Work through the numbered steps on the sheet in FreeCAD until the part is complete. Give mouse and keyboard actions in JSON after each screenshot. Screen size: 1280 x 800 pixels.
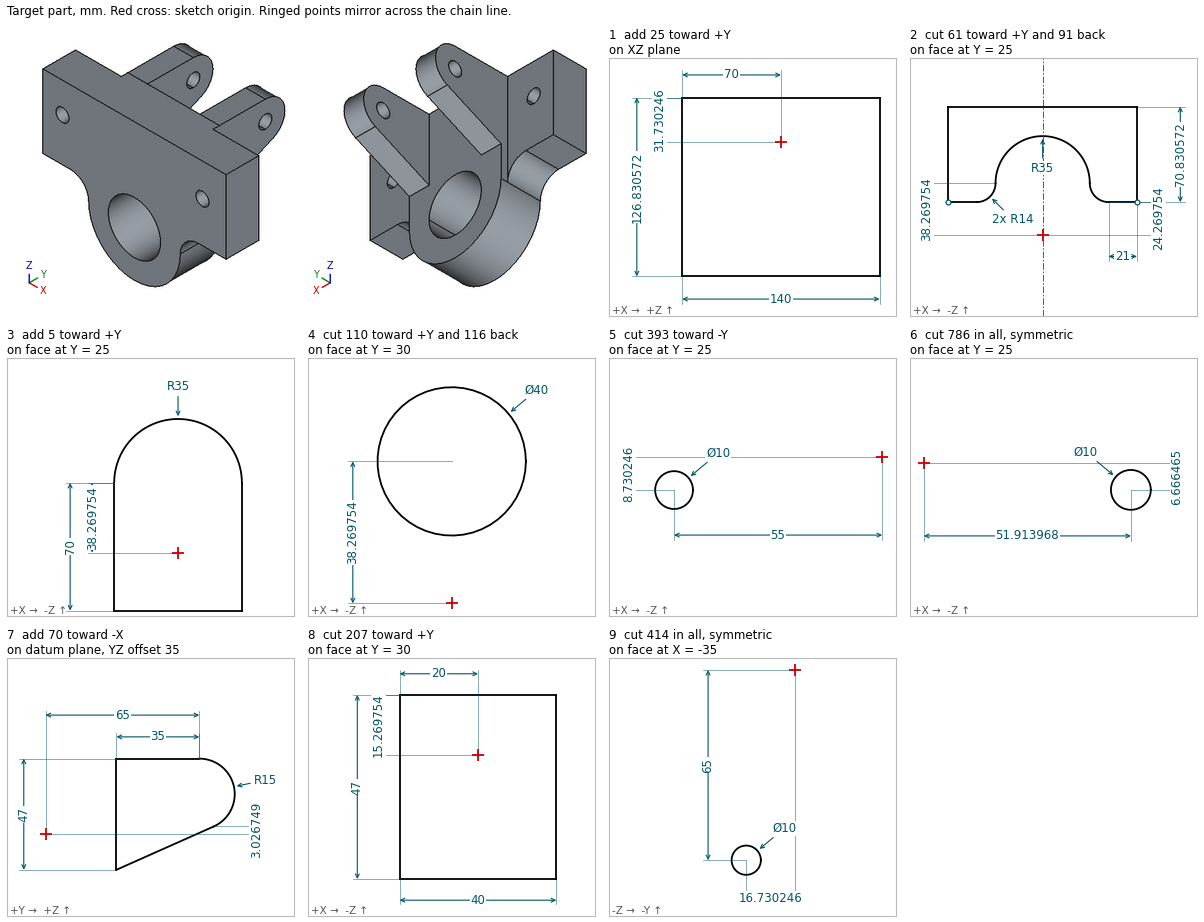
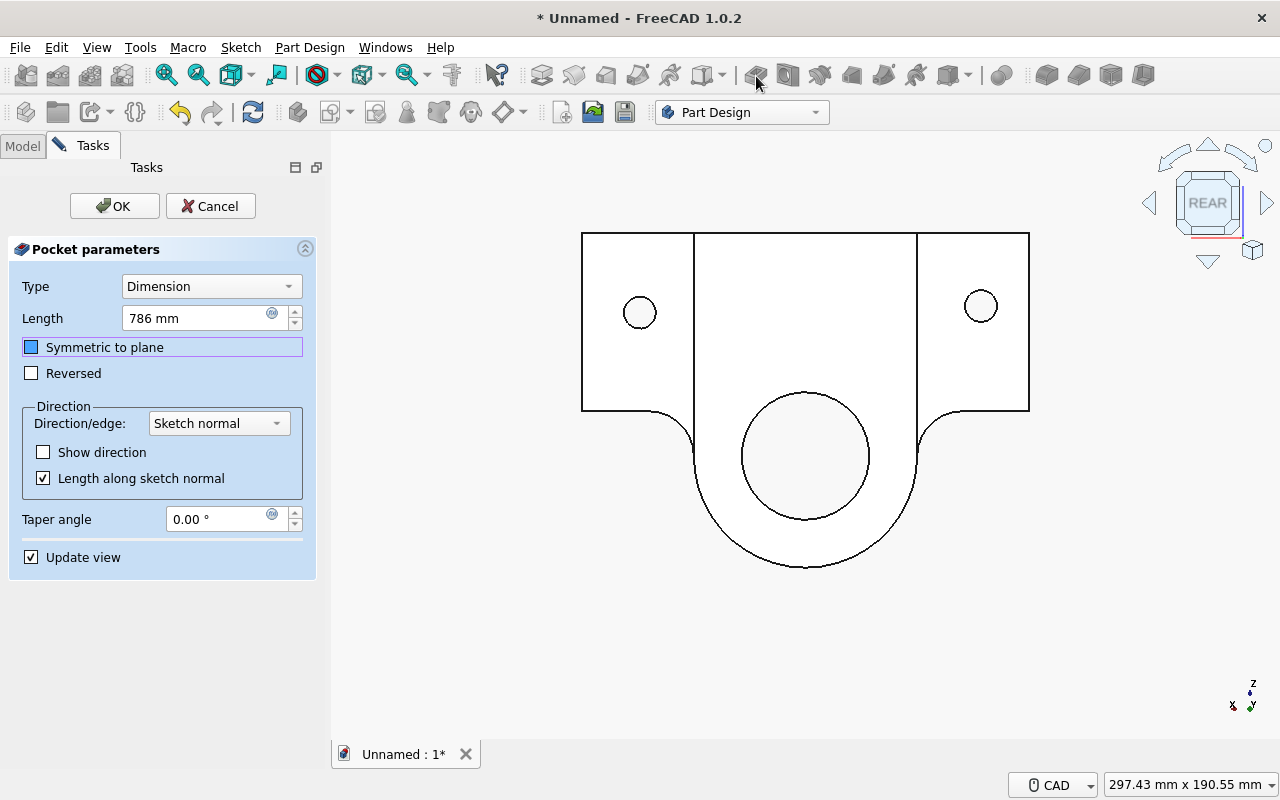
{"action": "left_click", "coordinate": [30, 347]}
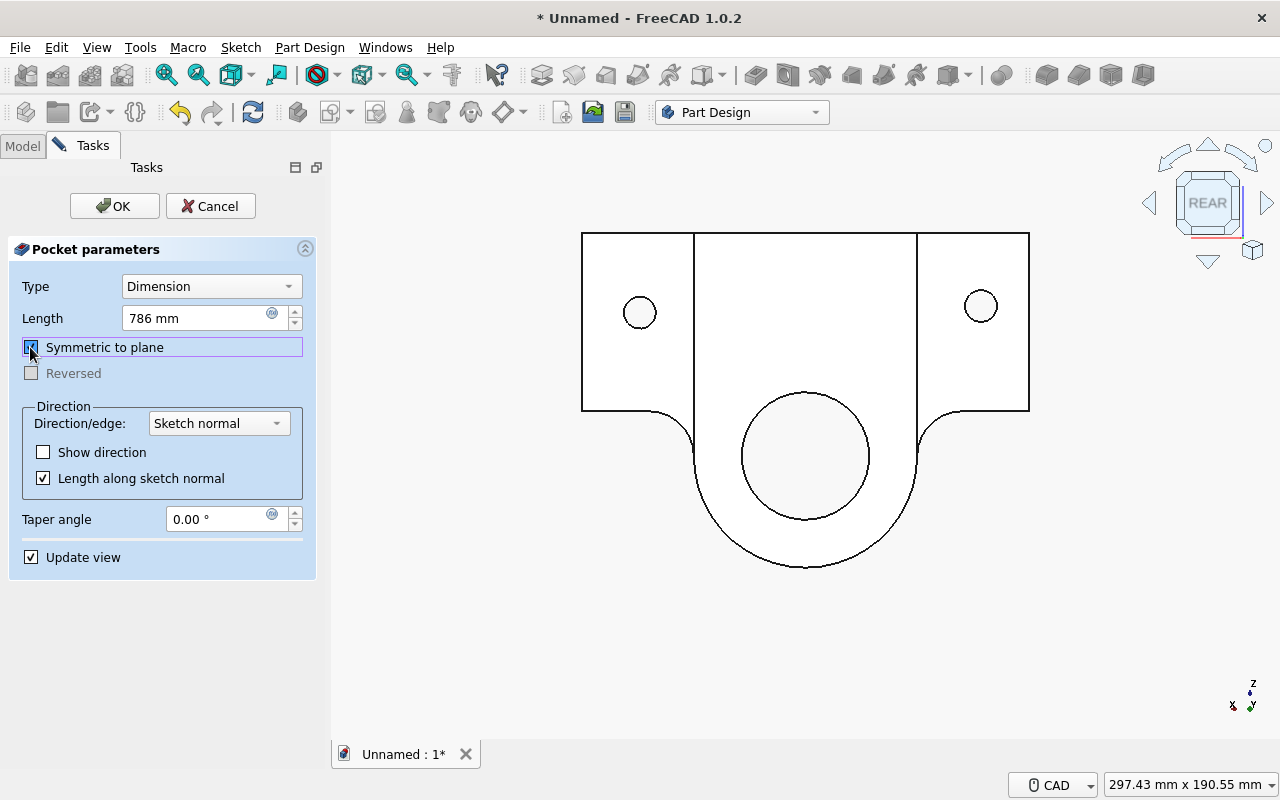
{"action": "left_click", "coordinate": [115, 206]}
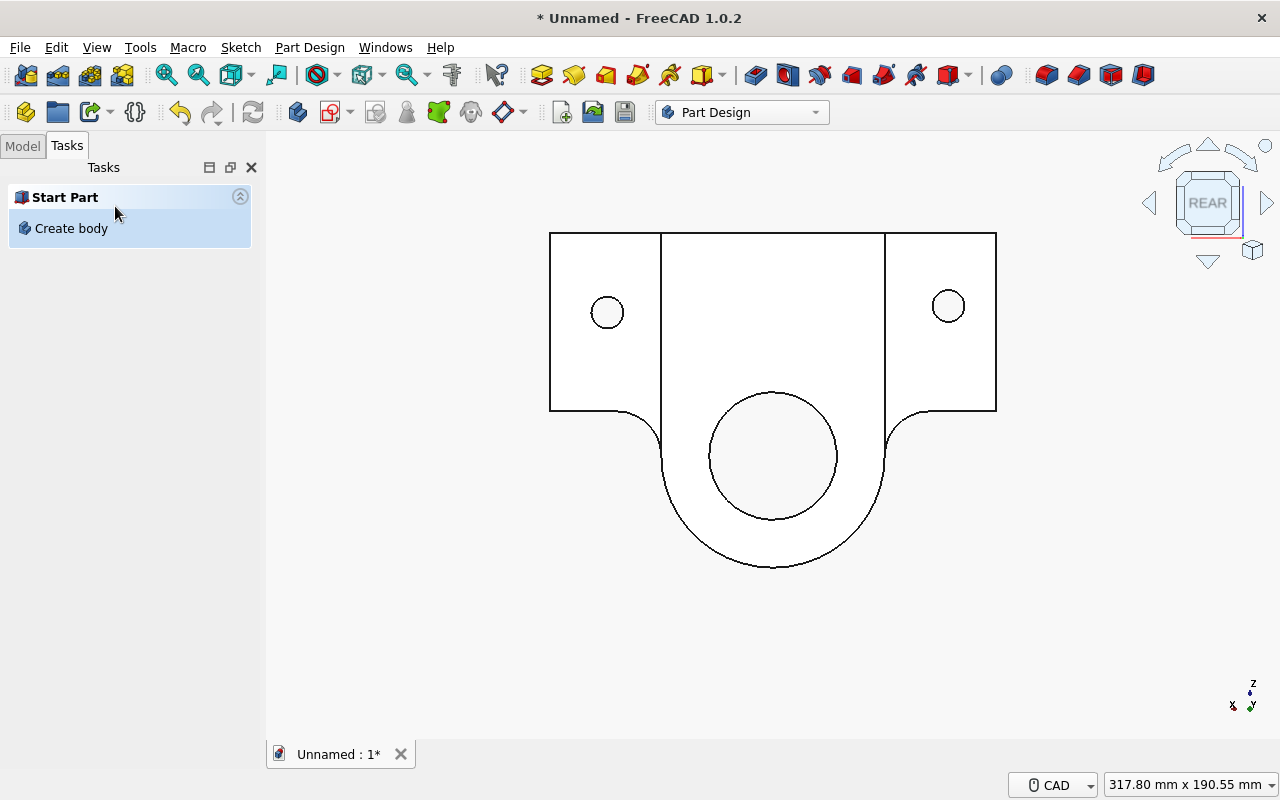
{"action": "key", "text": "0"}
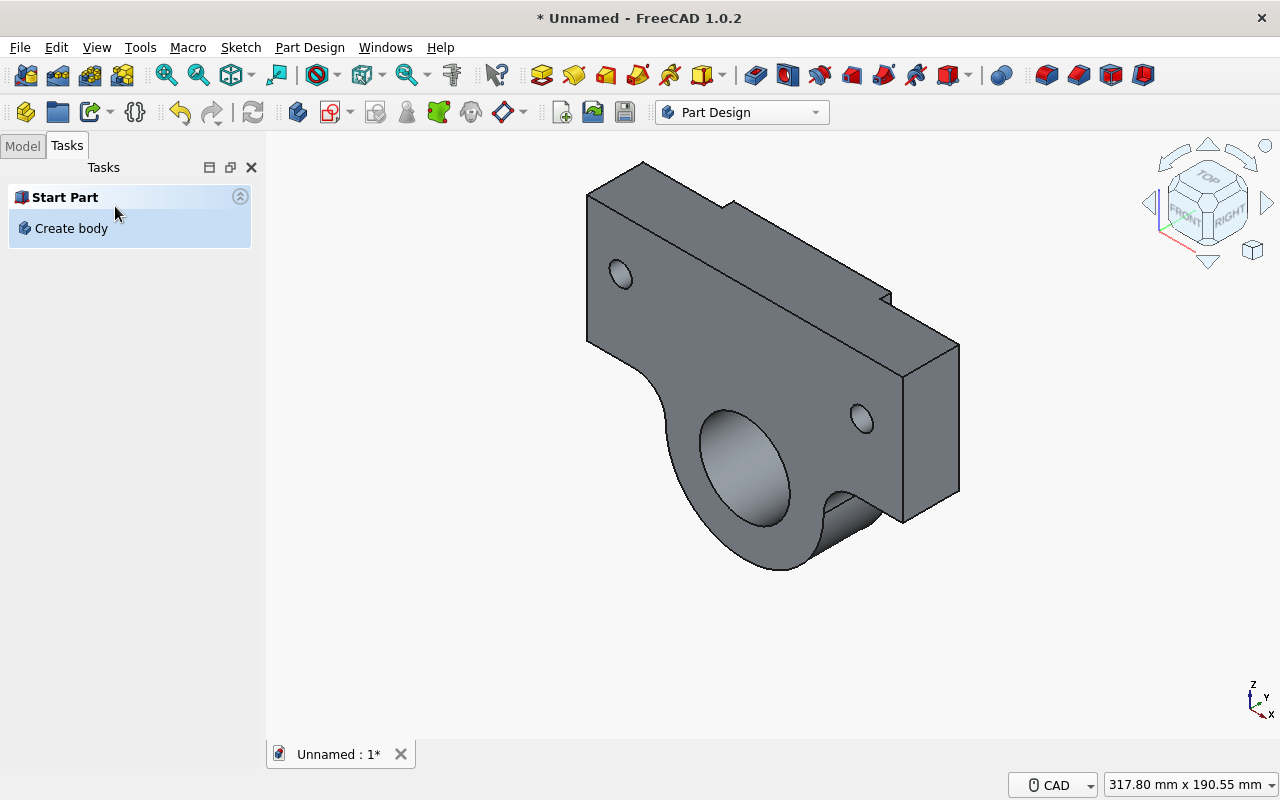
{"action": "key", "text": "3"}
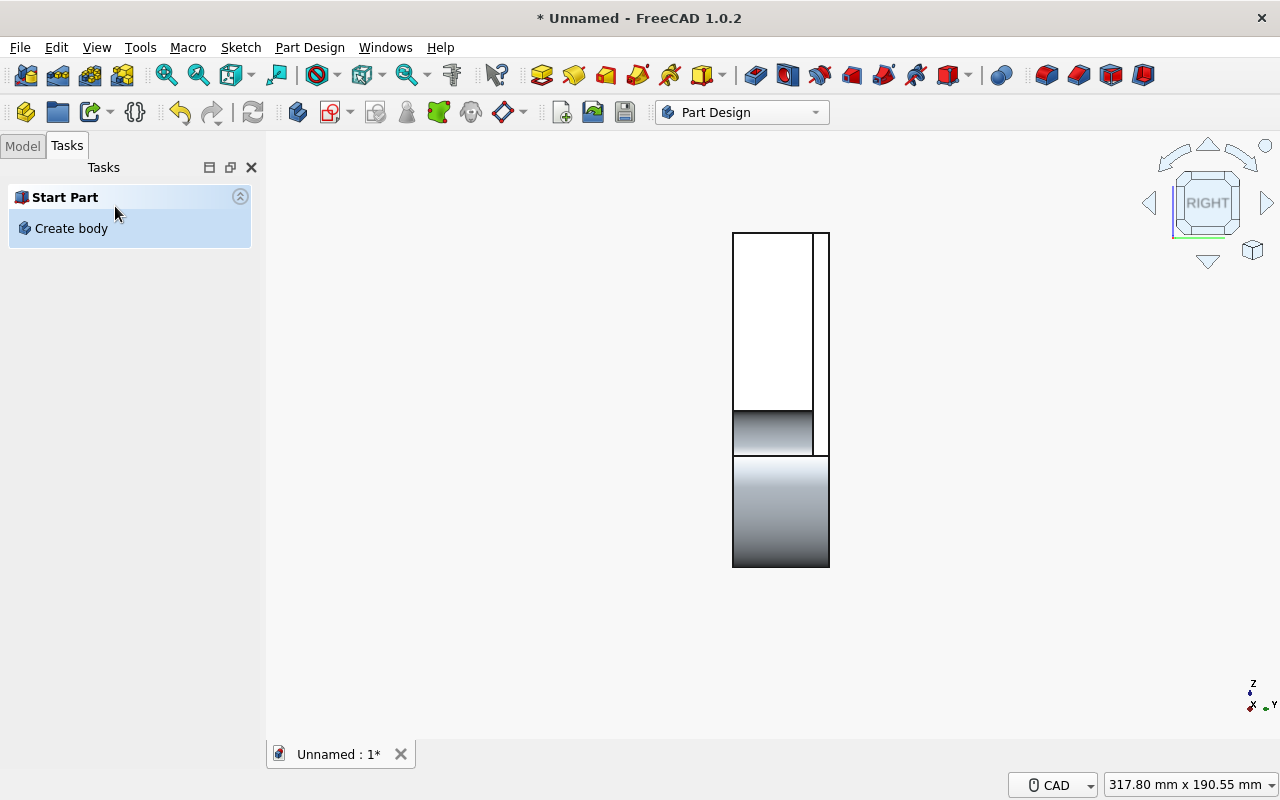
{"action": "key", "text": "2"}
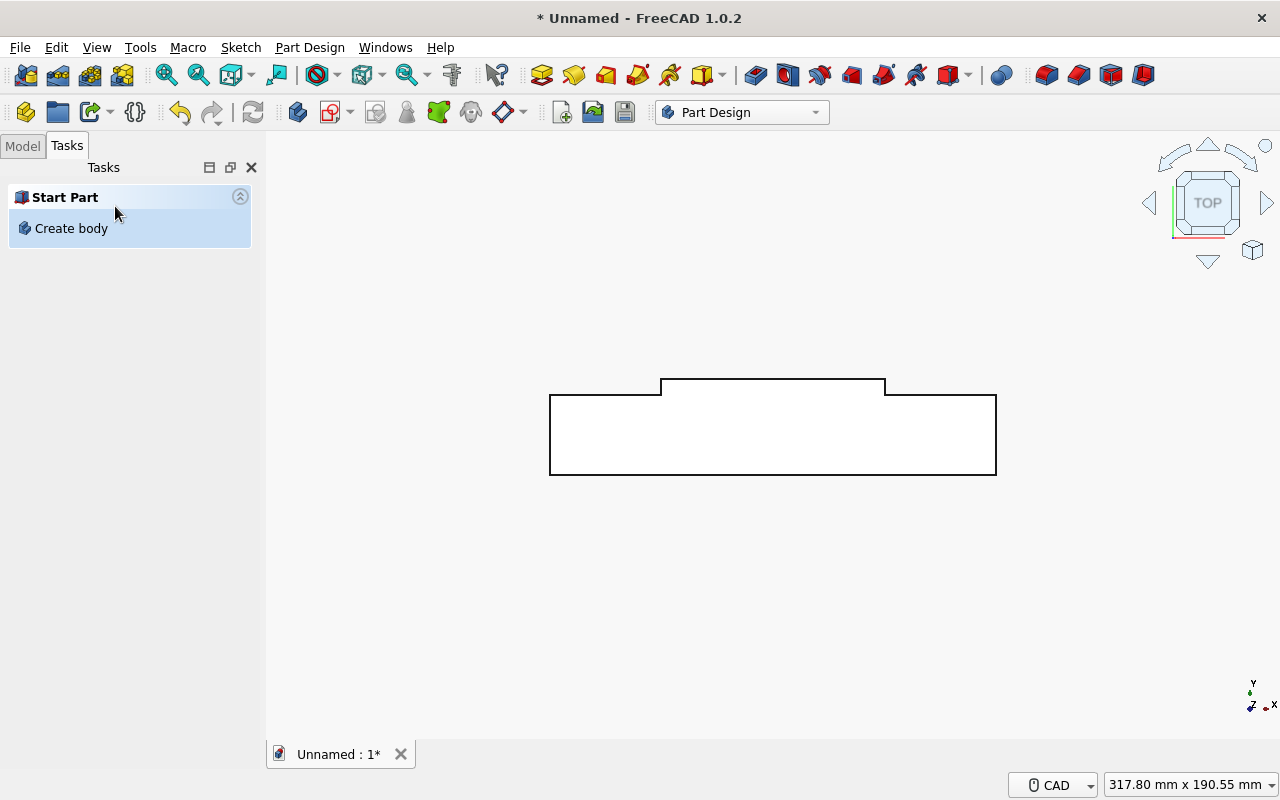
{"action": "left_click", "coordinate": [168, 76]}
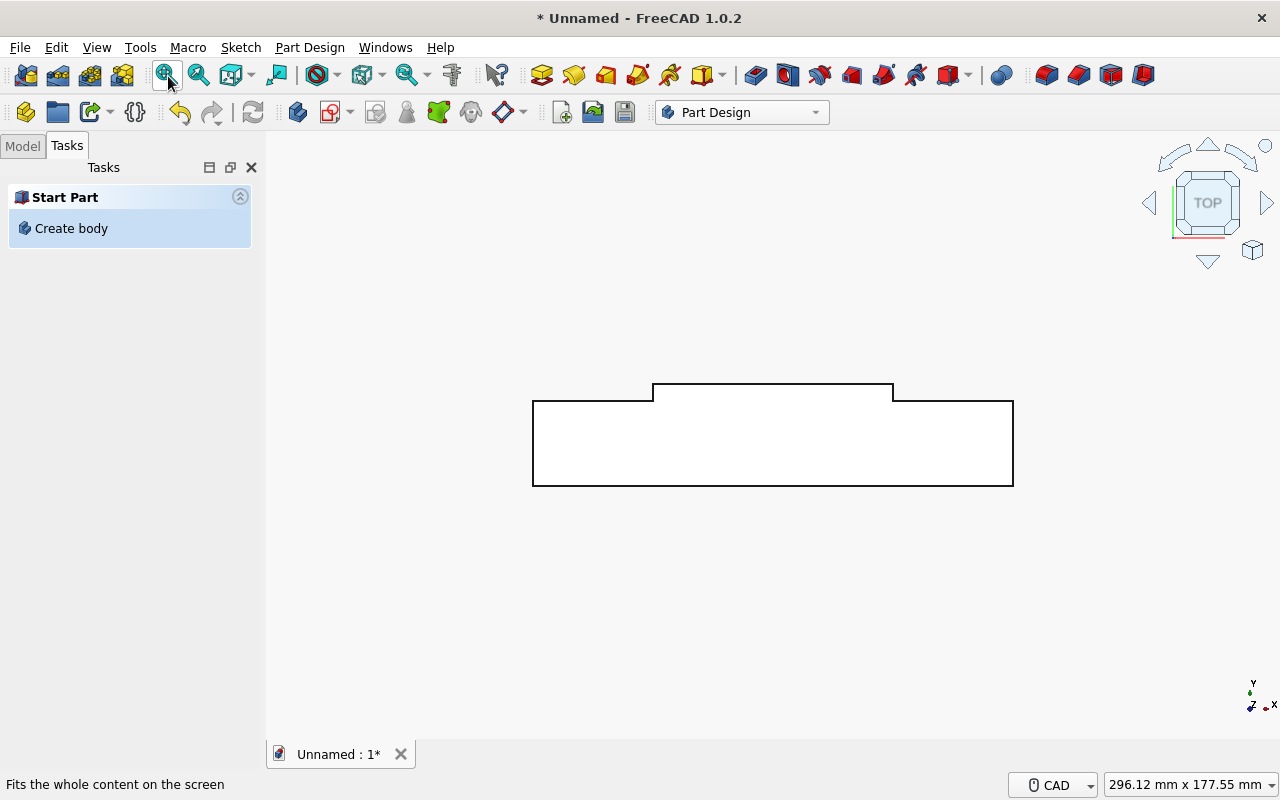
{"action": "left_click", "coordinate": [23, 145]}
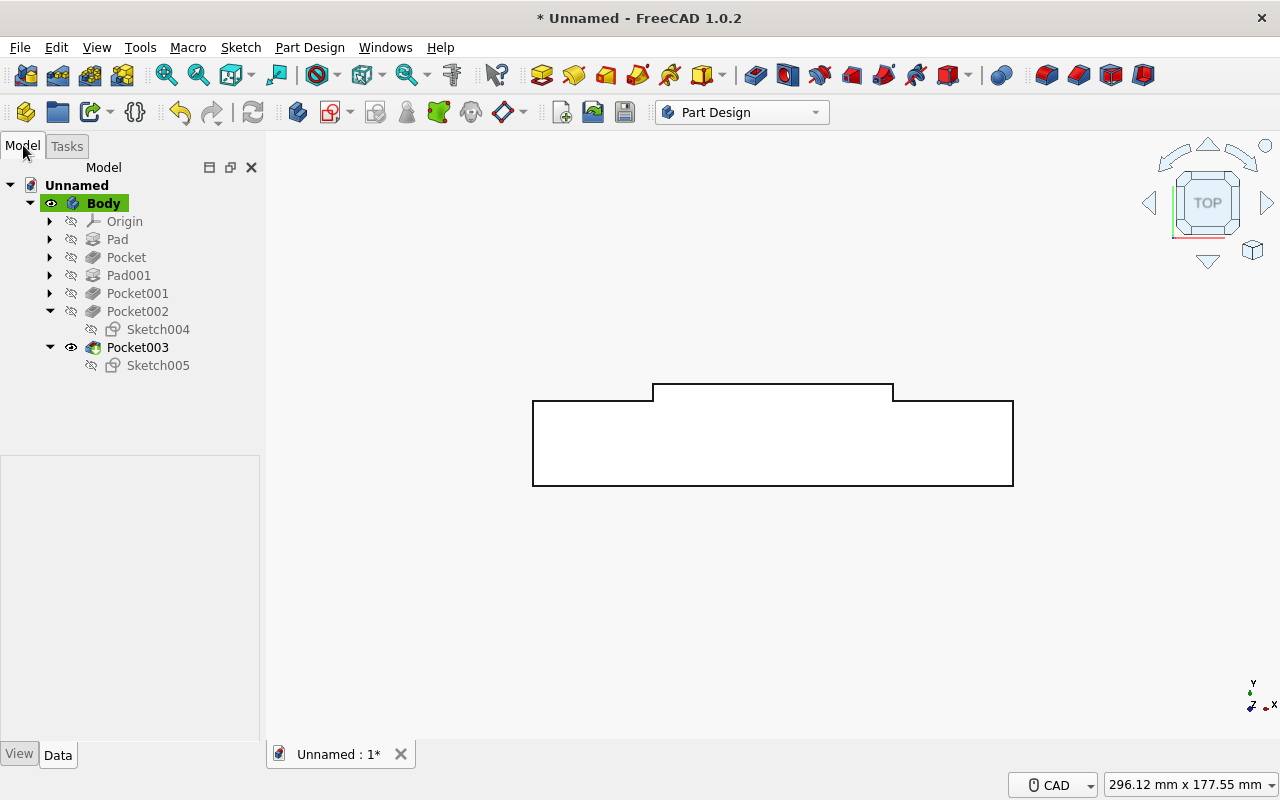
{"action": "left_click", "coordinate": [50, 221]}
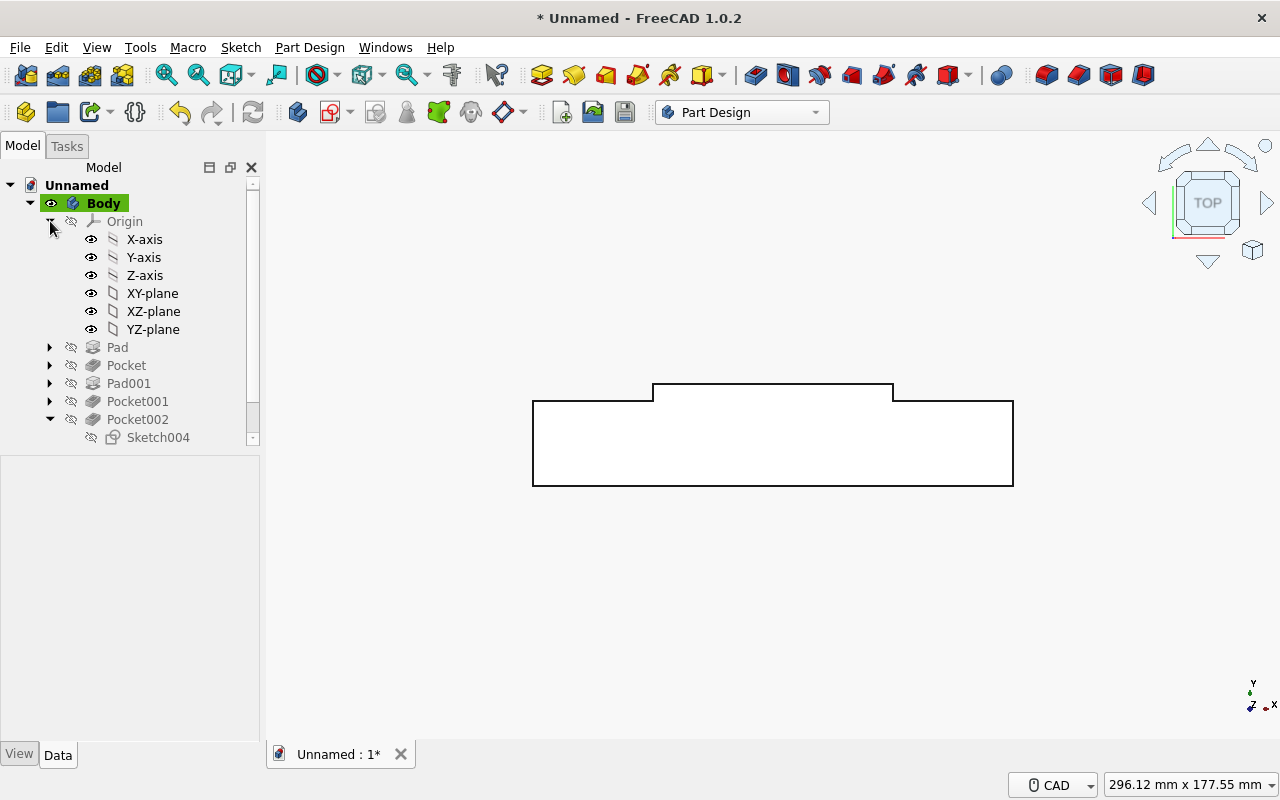
{"action": "left_click", "coordinate": [136, 329]}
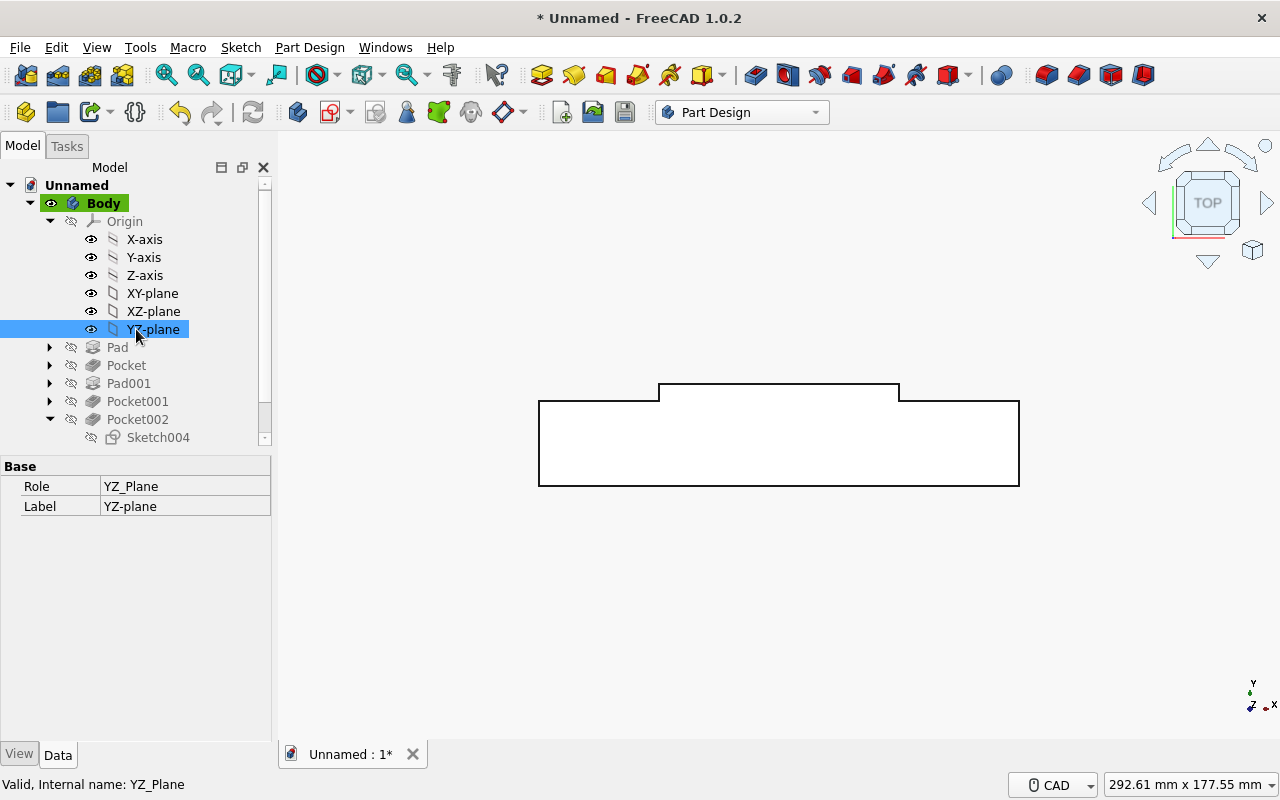
{"action": "left_click", "coordinate": [504, 112]}